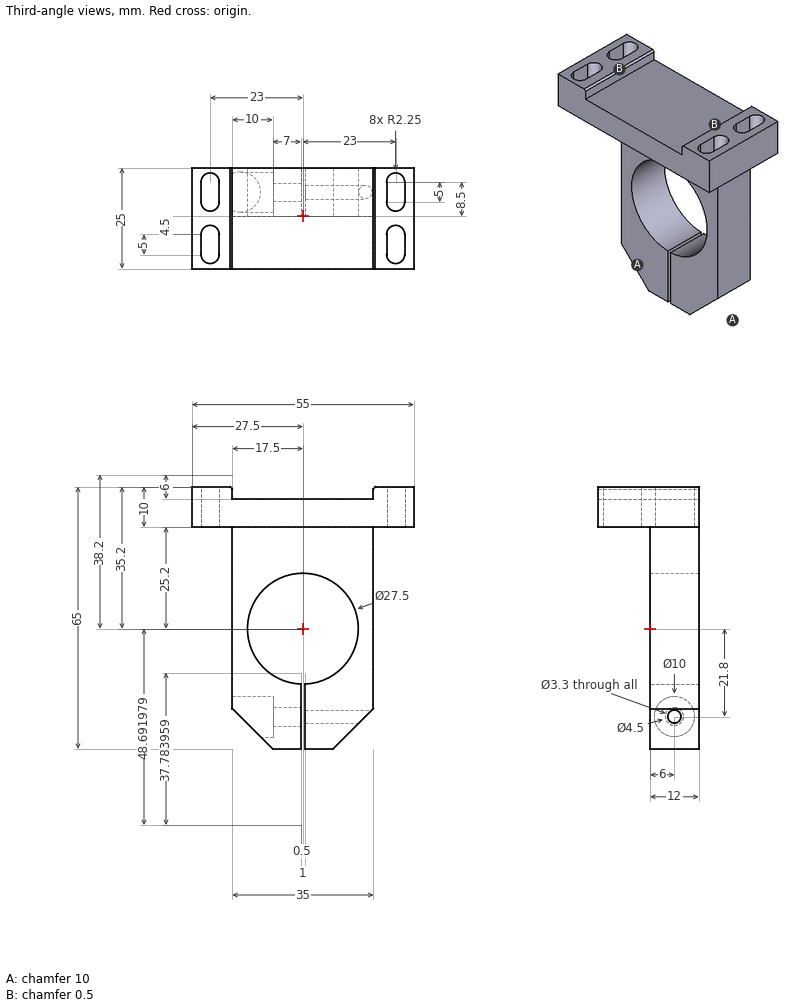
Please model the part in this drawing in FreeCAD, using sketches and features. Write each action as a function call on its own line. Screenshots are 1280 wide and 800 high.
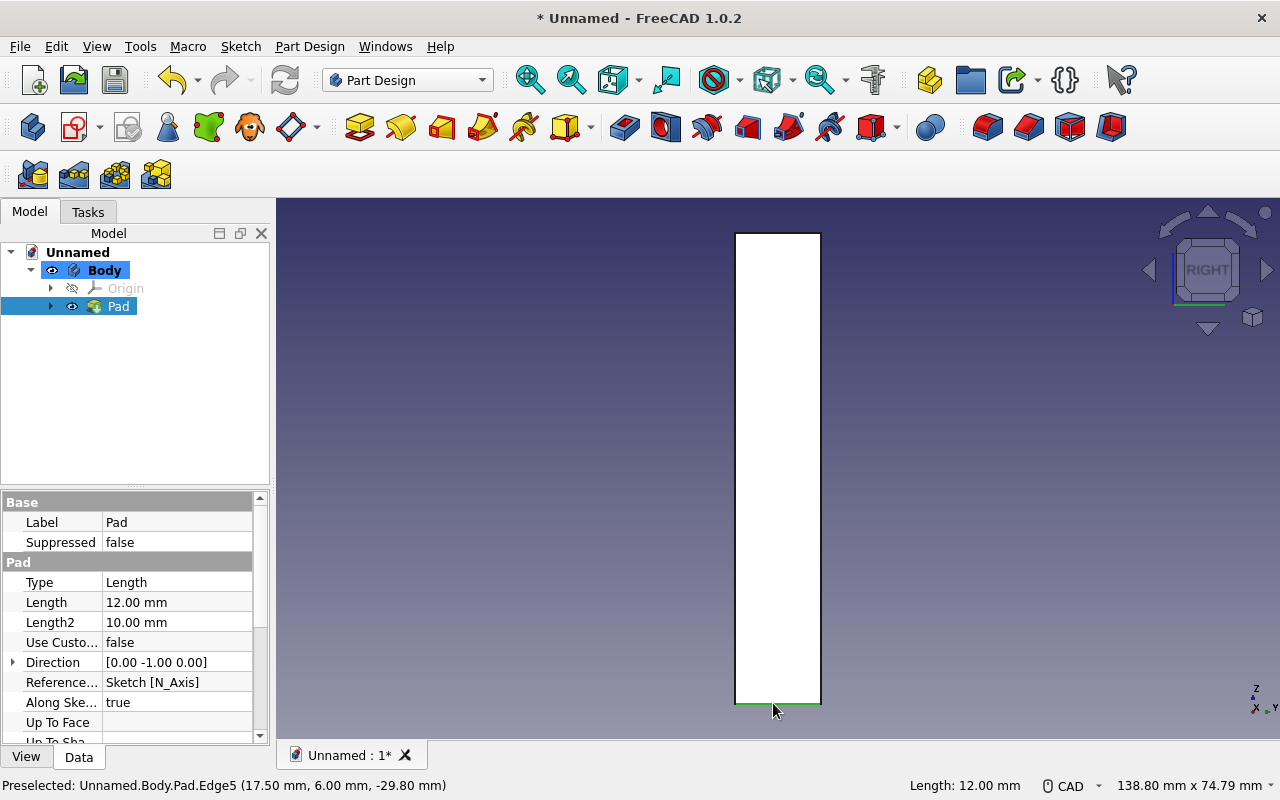
key(5)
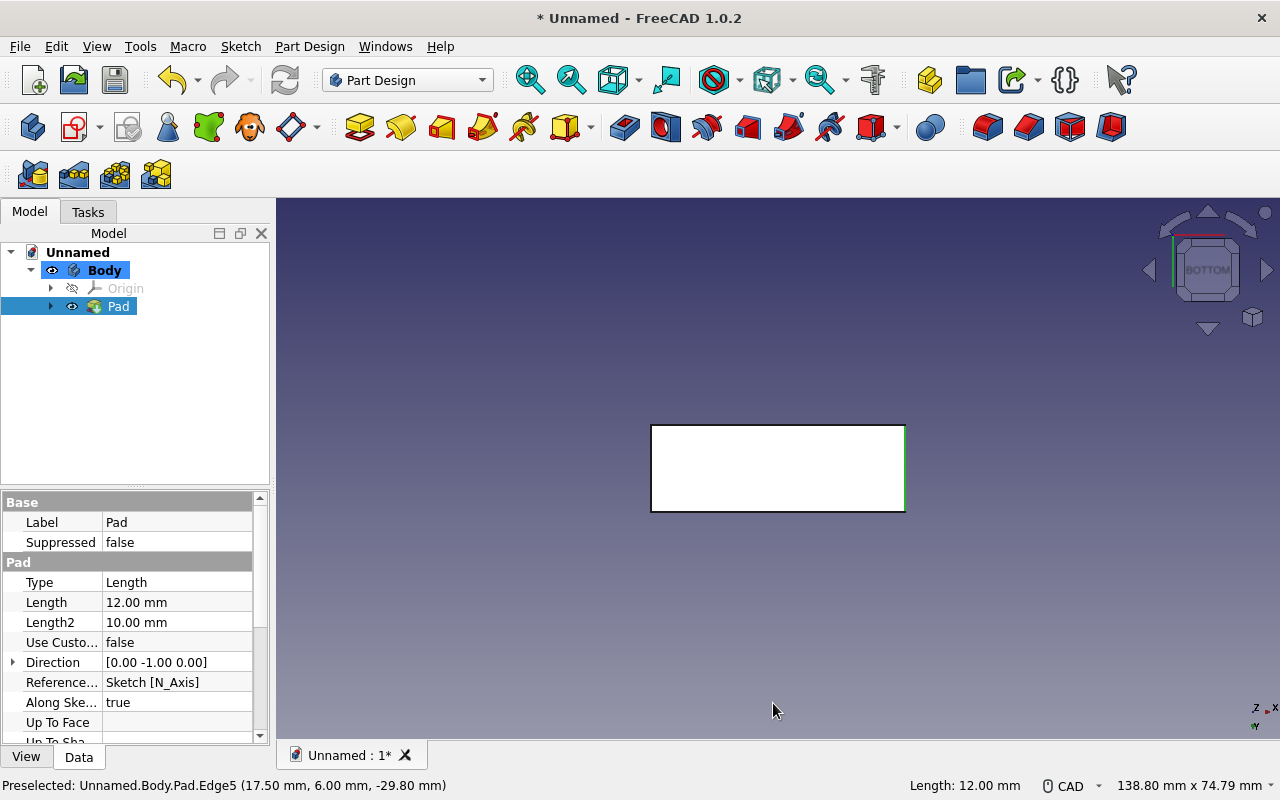
key(v)
key(f)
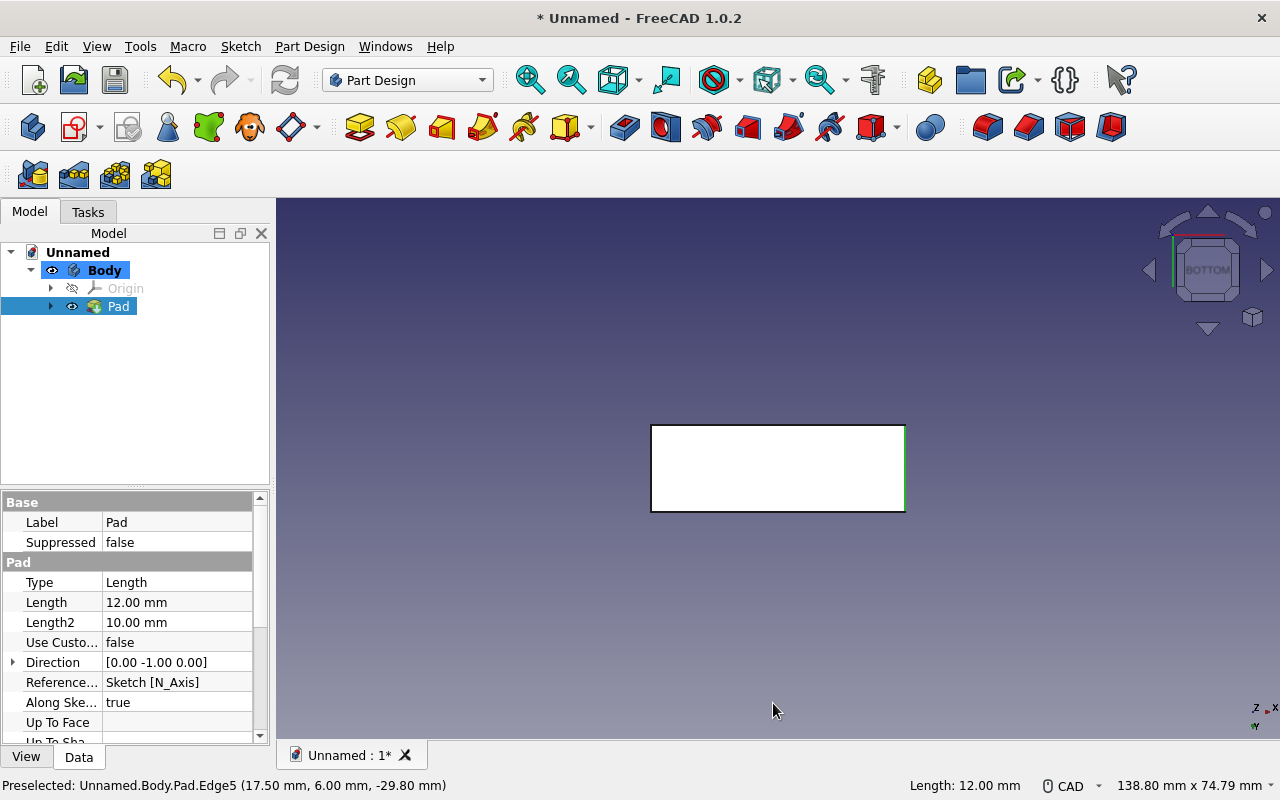
click(651, 467, ctrl)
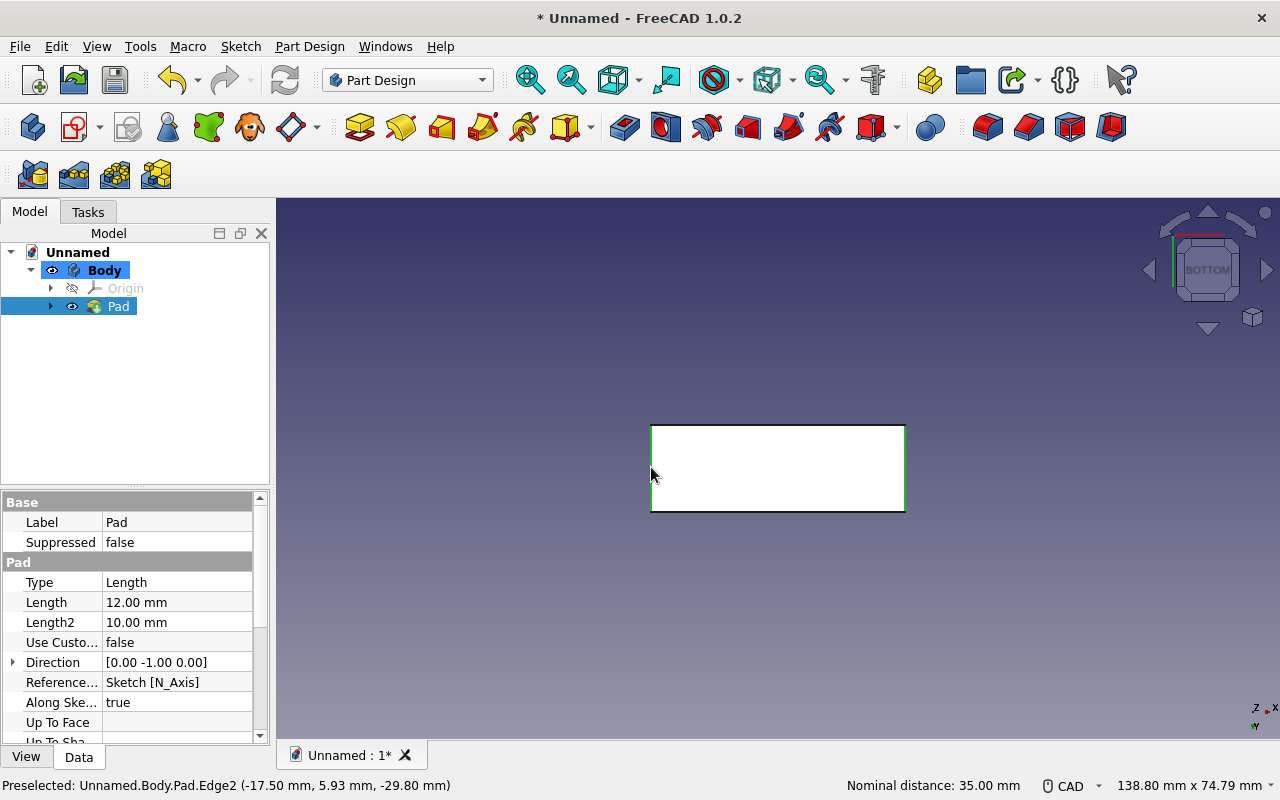
click(1029, 128)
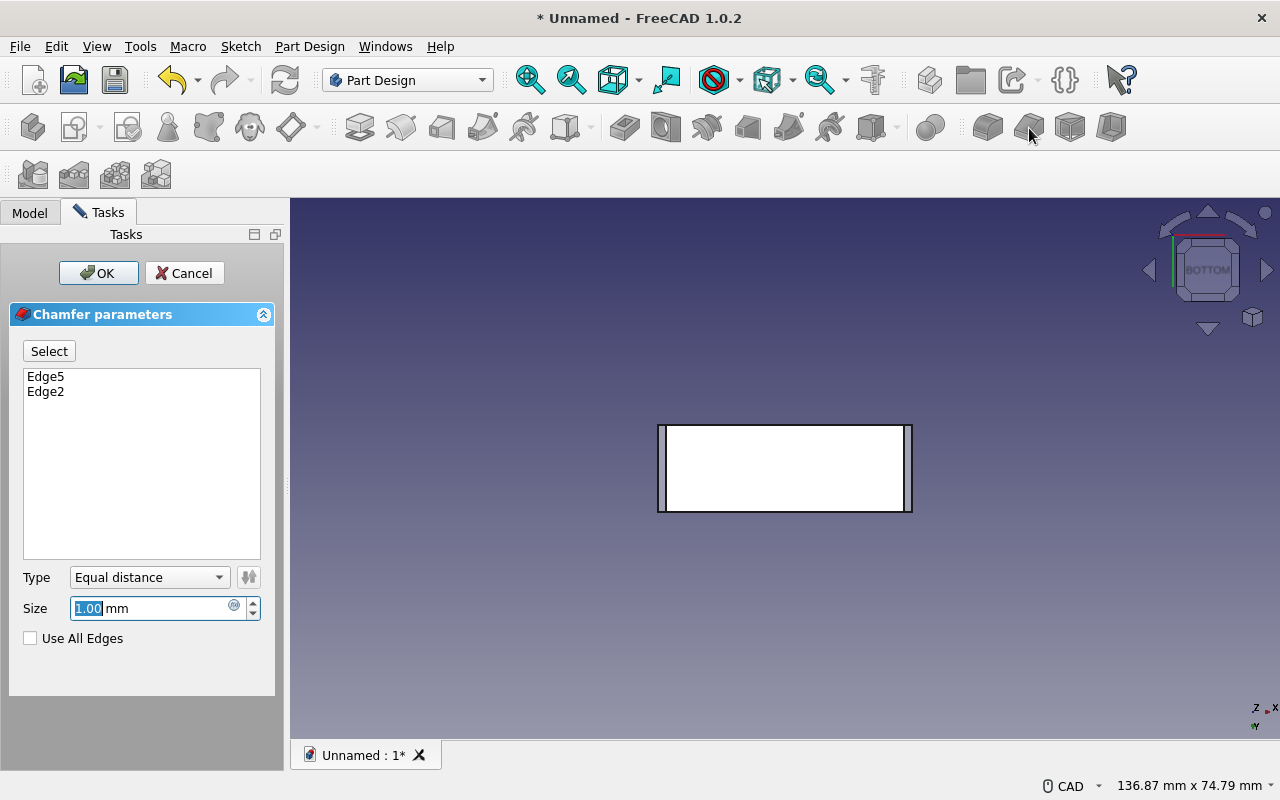
text(10)
key(Tab)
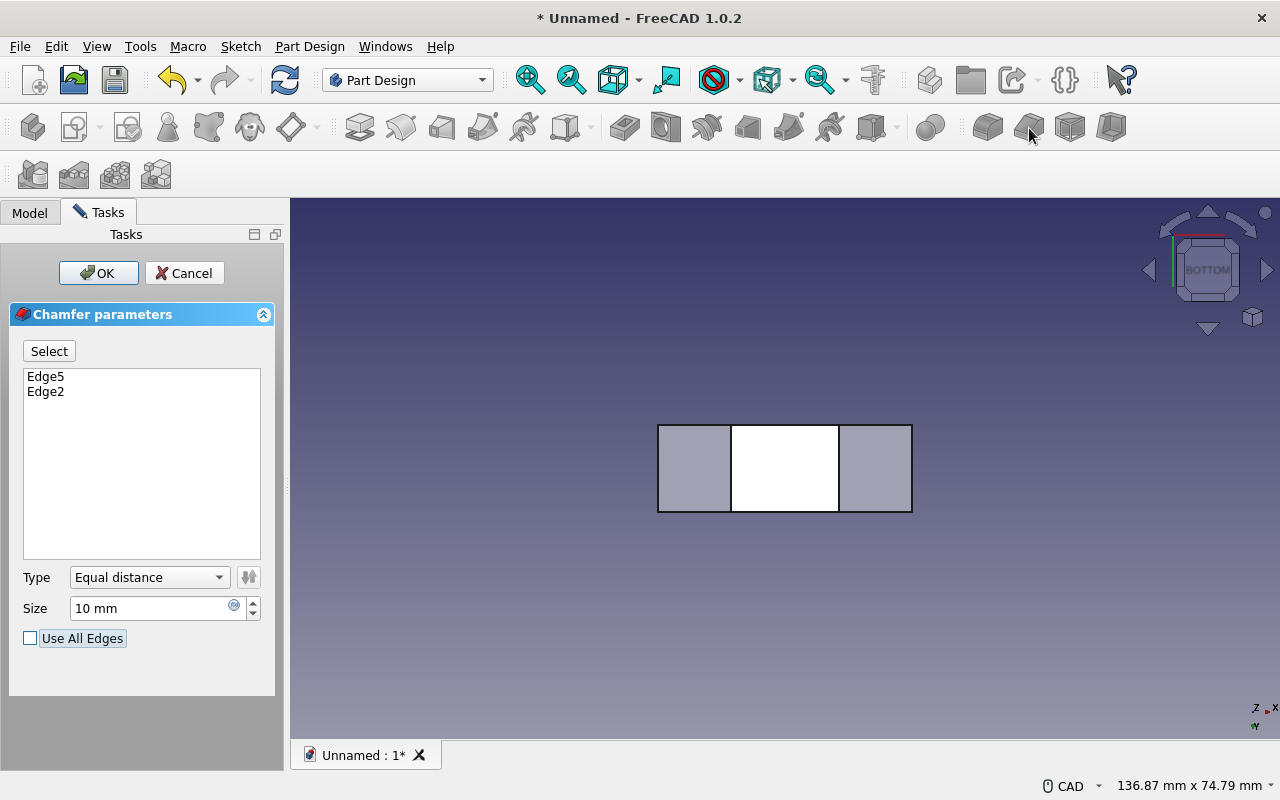
click(99, 273)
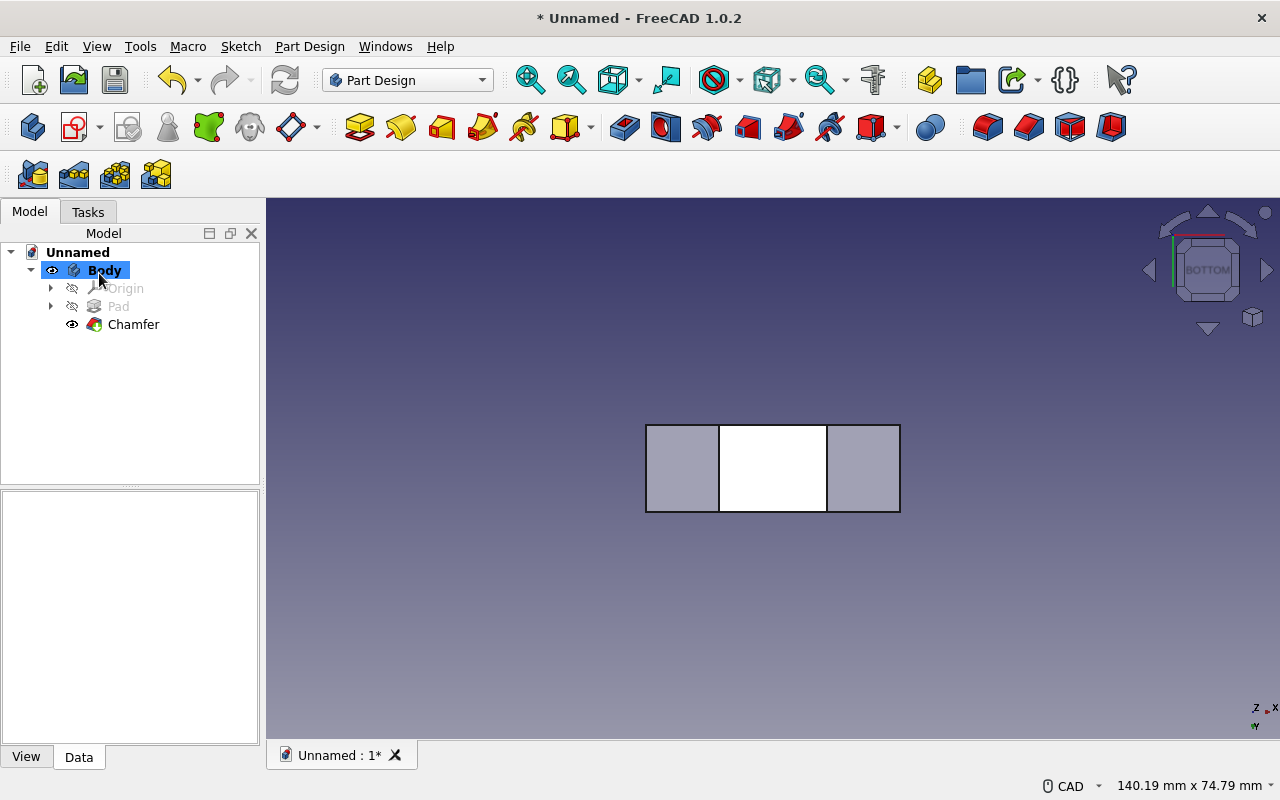
key(v)
key(f)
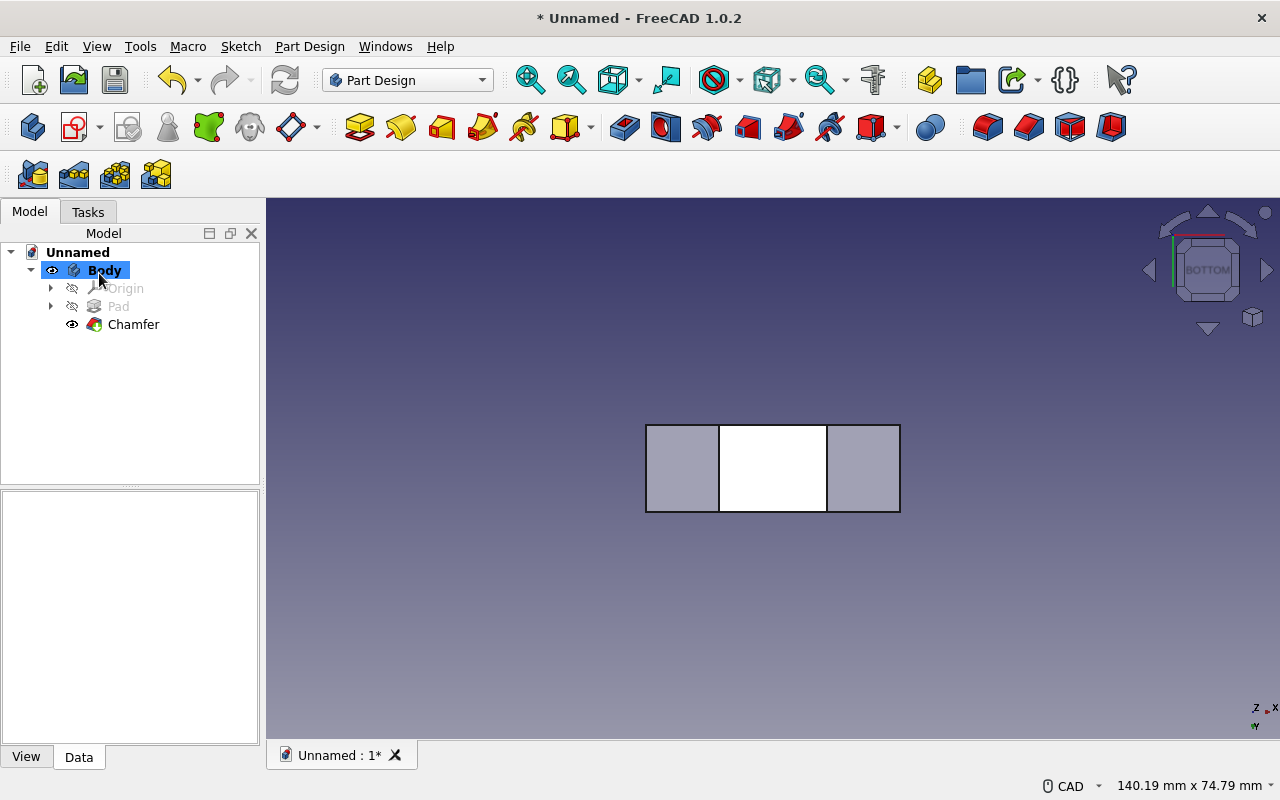
key(4)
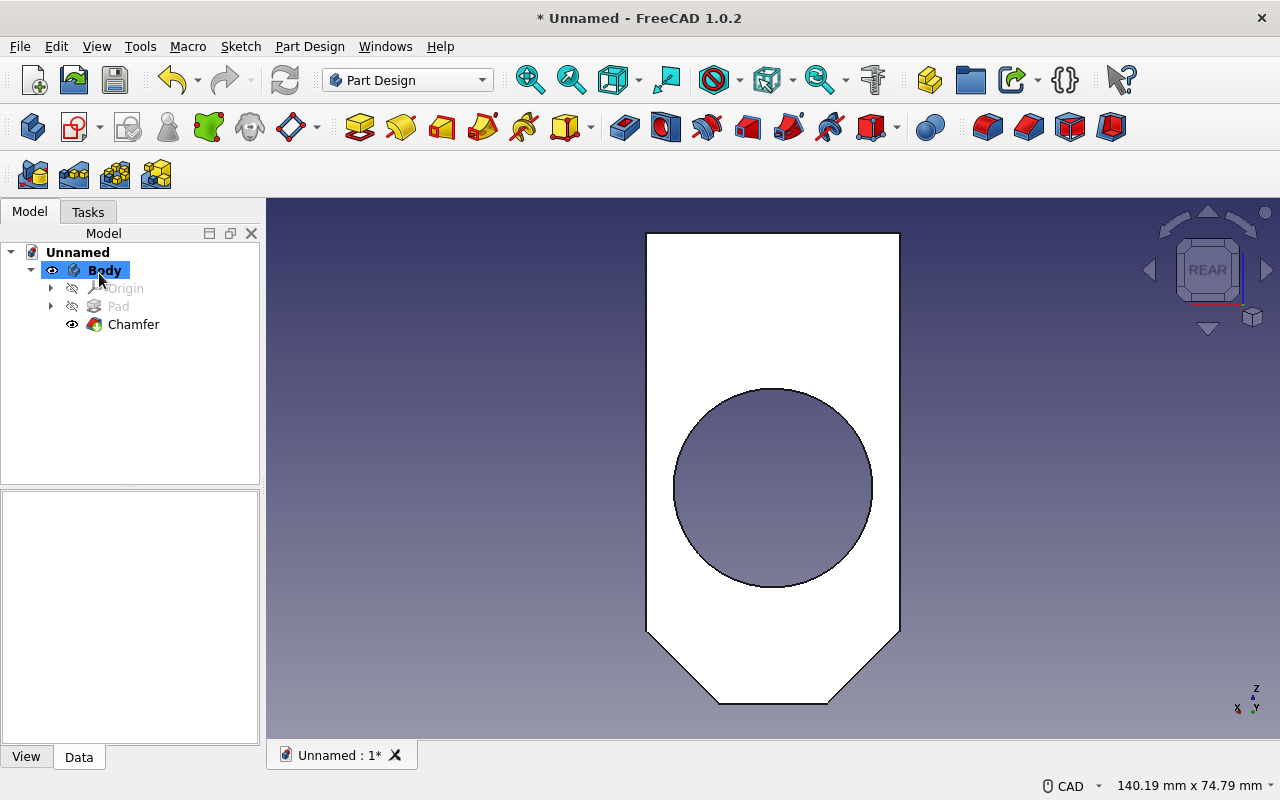
click(809, 333)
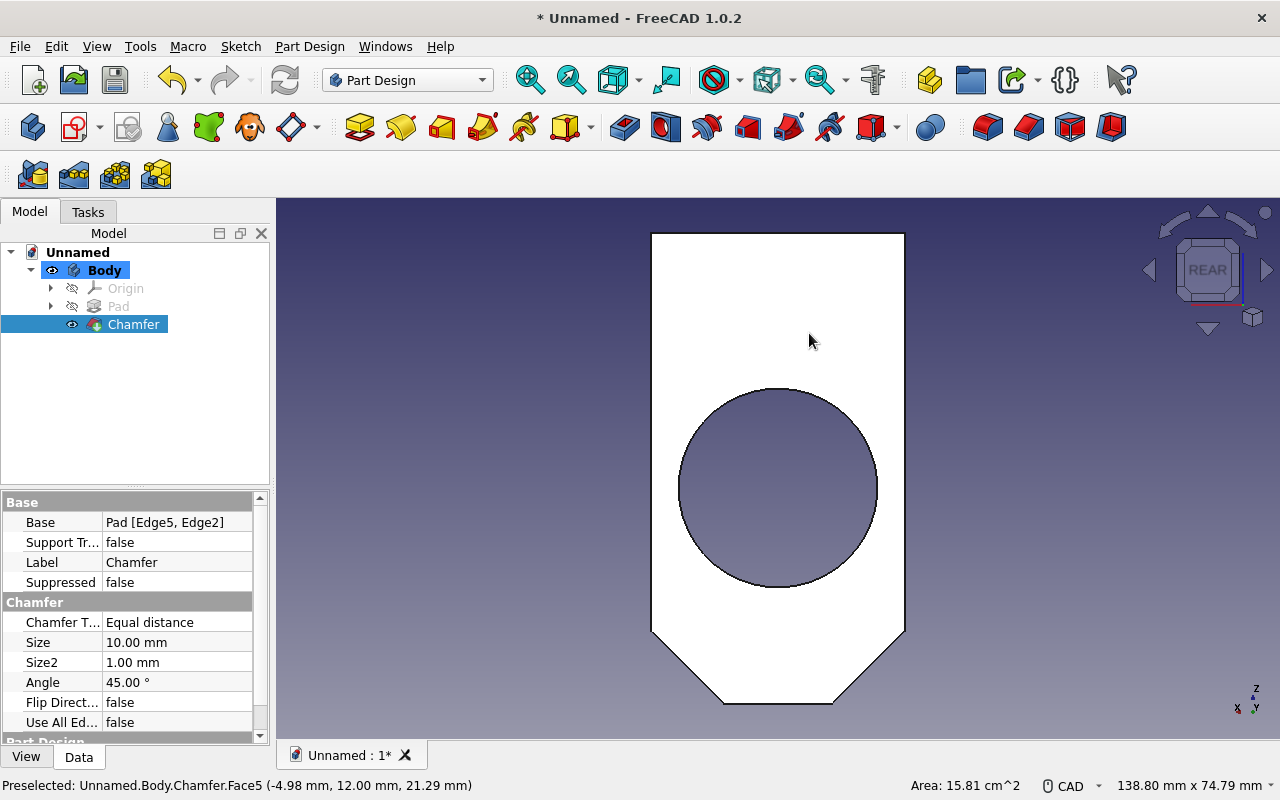
click(74, 128)